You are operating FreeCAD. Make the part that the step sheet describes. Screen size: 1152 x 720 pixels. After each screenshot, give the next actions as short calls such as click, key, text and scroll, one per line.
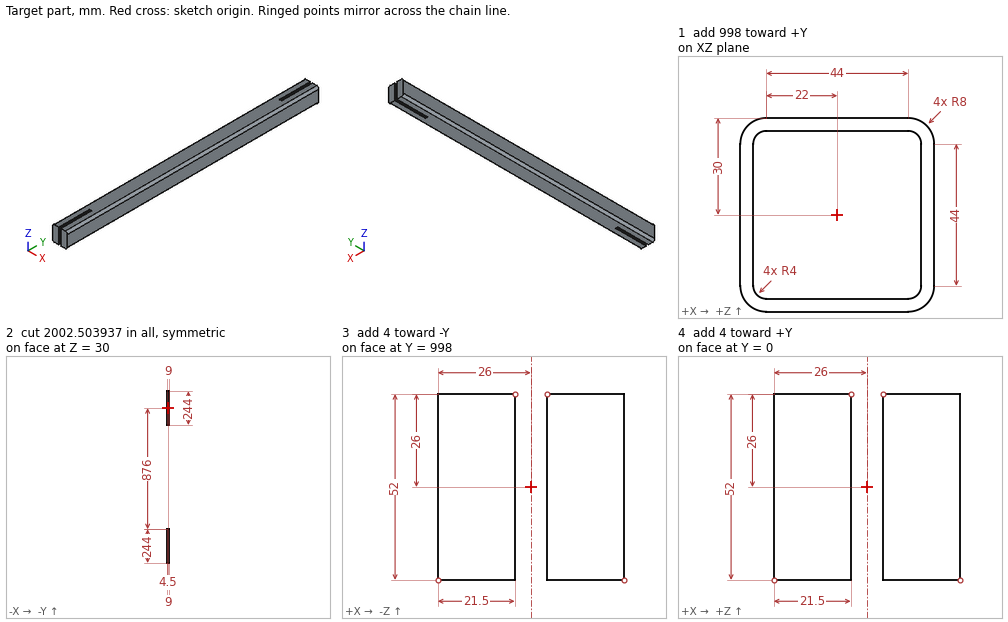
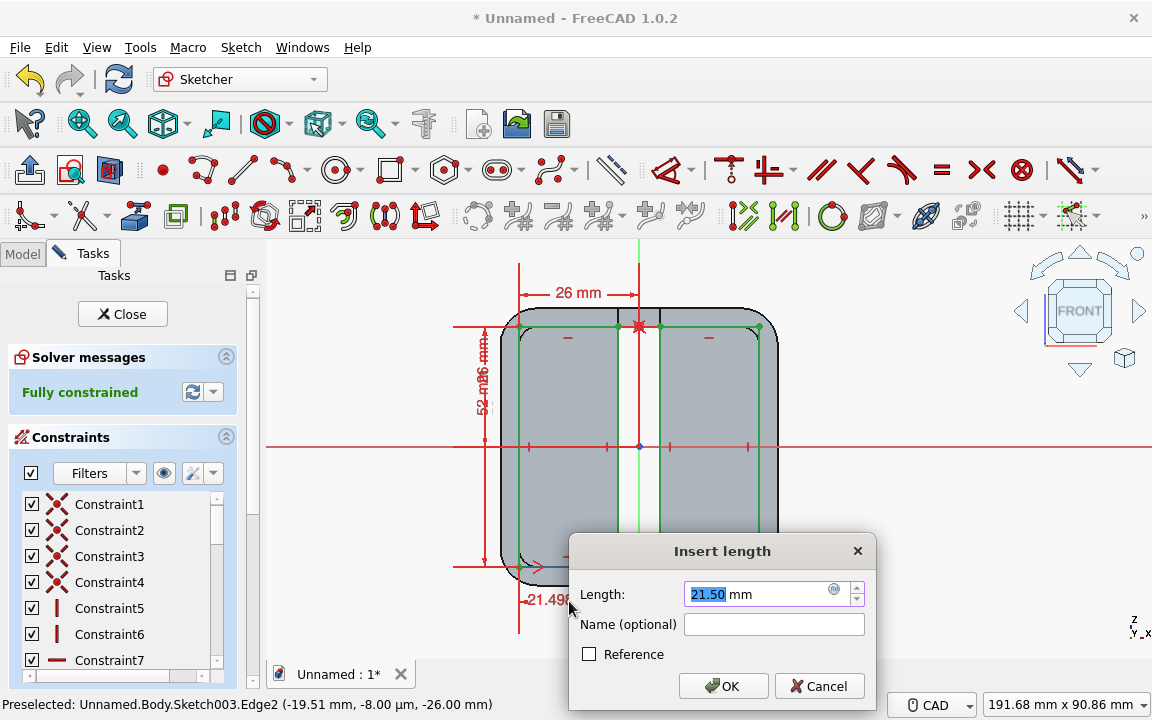
text(21.5)
key(Return)
key(Escape)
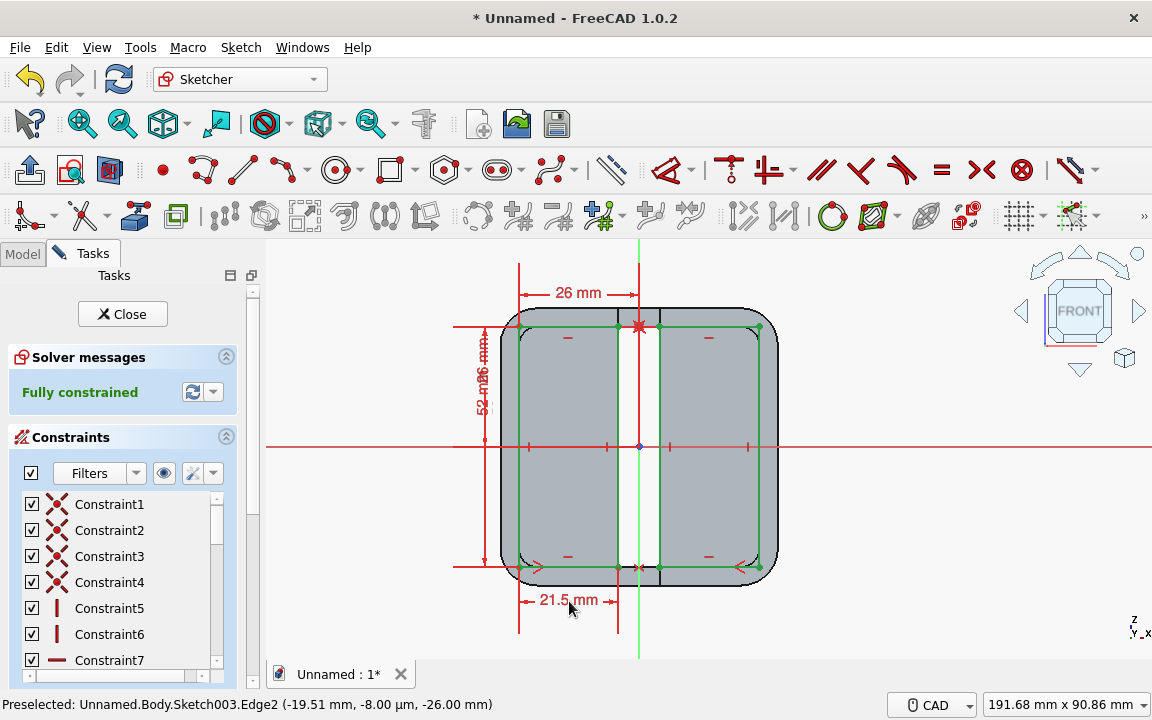
click(123, 314)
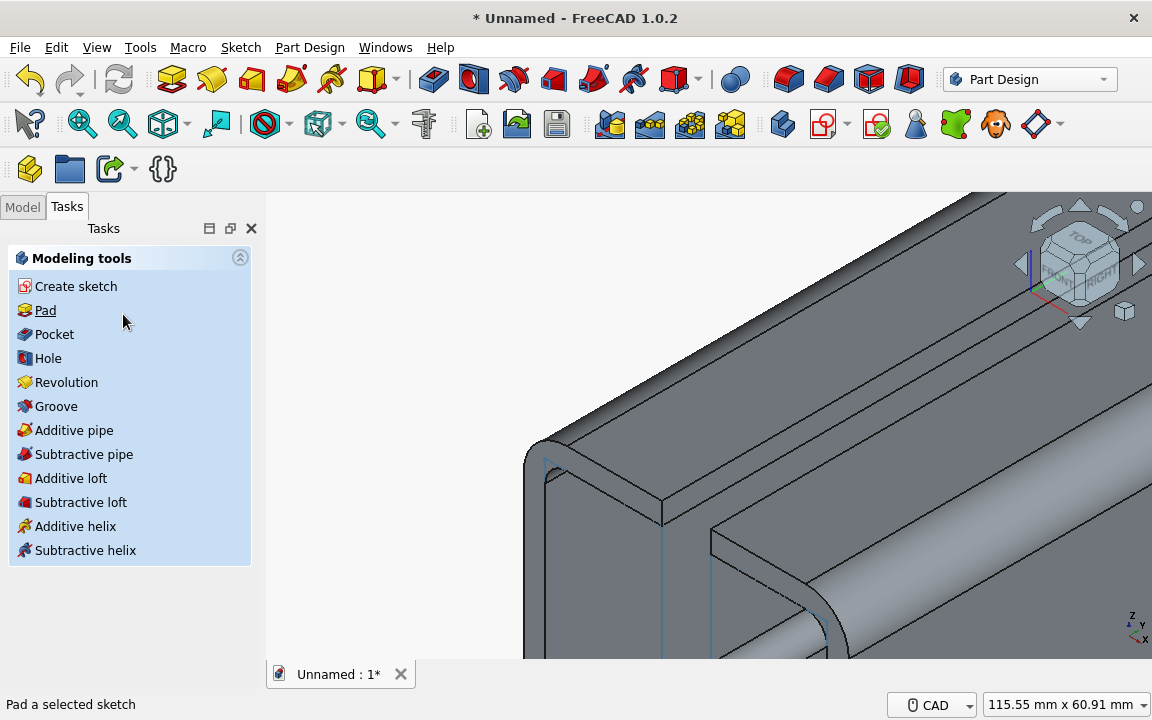
click(172, 80)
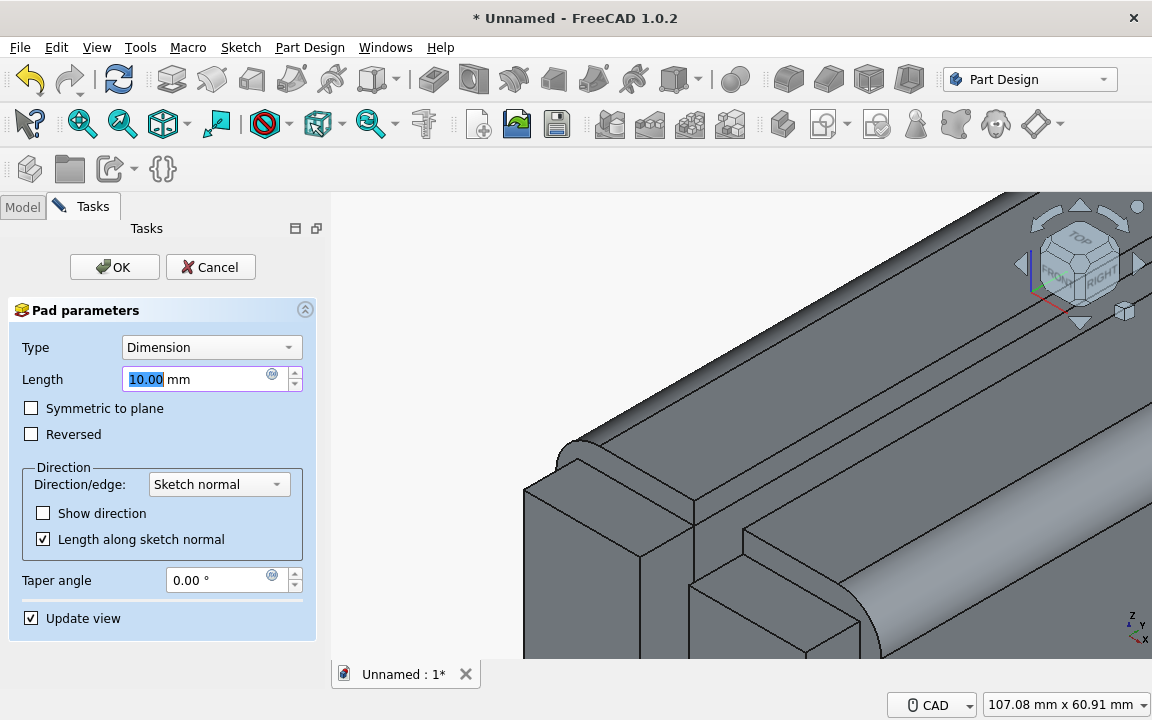
text(4)
key(Tab)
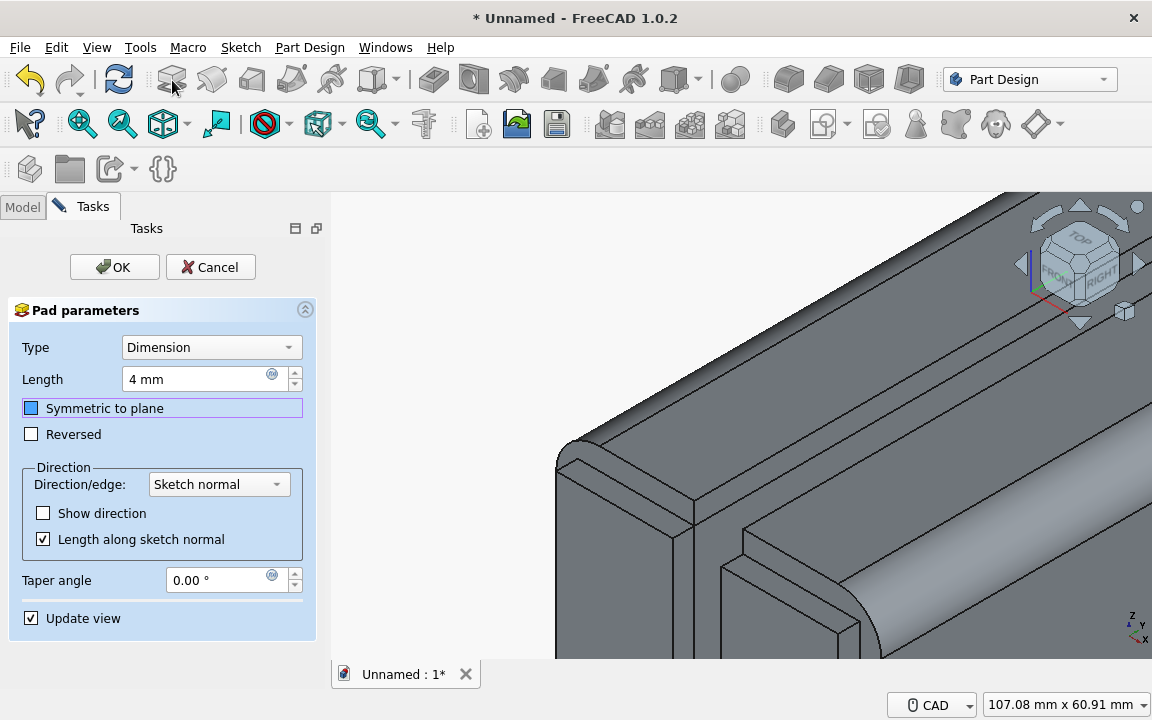
click(30, 434)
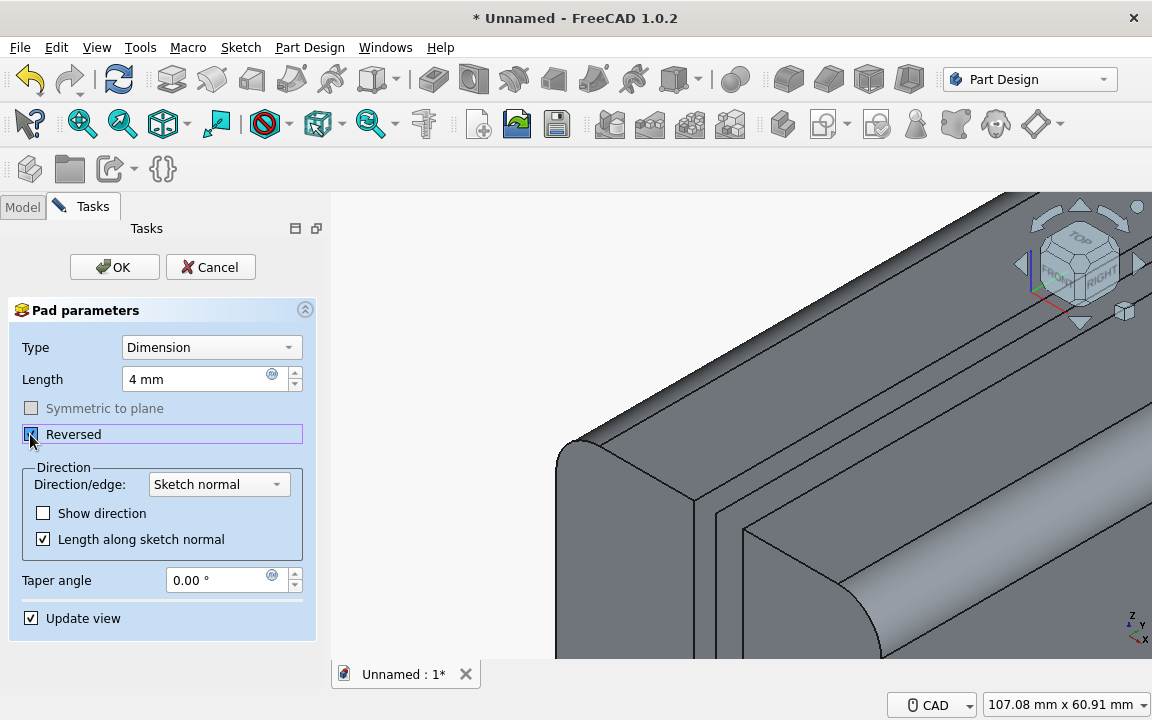
click(115, 267)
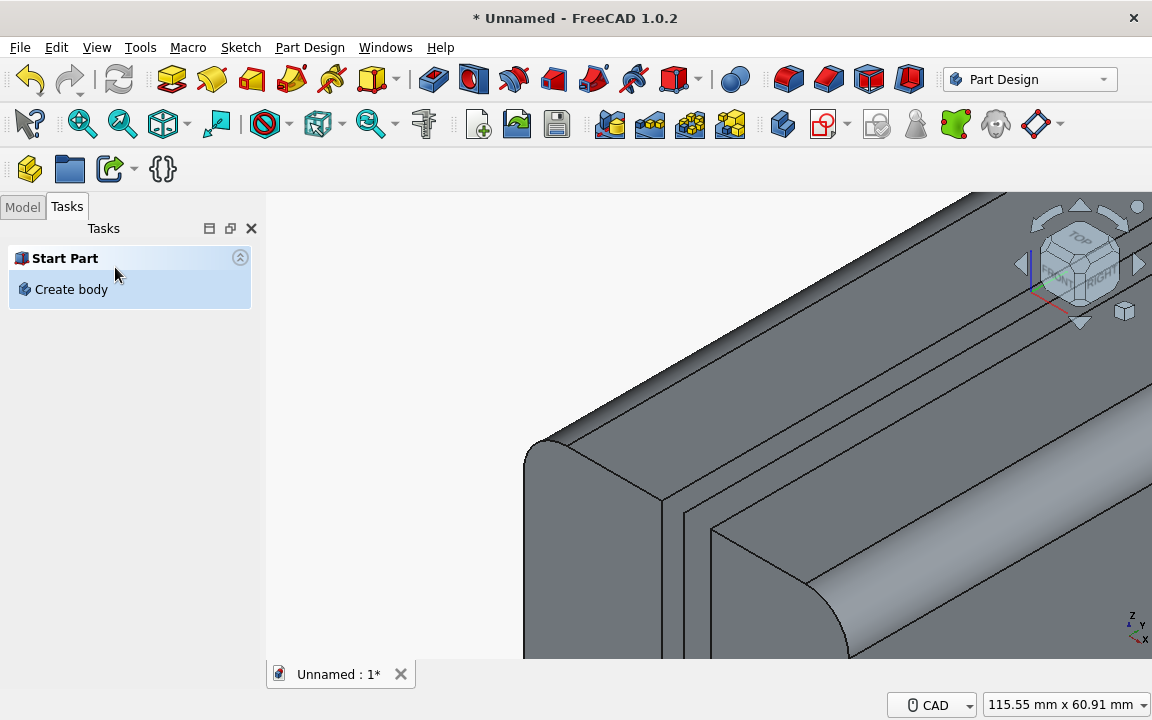
click(84, 124)